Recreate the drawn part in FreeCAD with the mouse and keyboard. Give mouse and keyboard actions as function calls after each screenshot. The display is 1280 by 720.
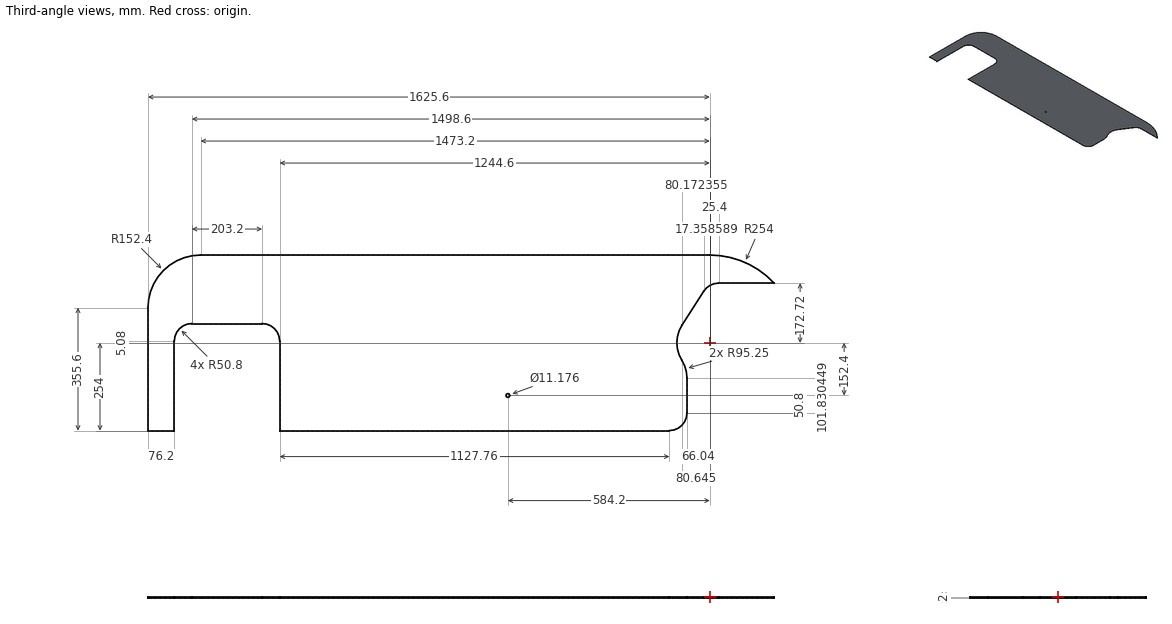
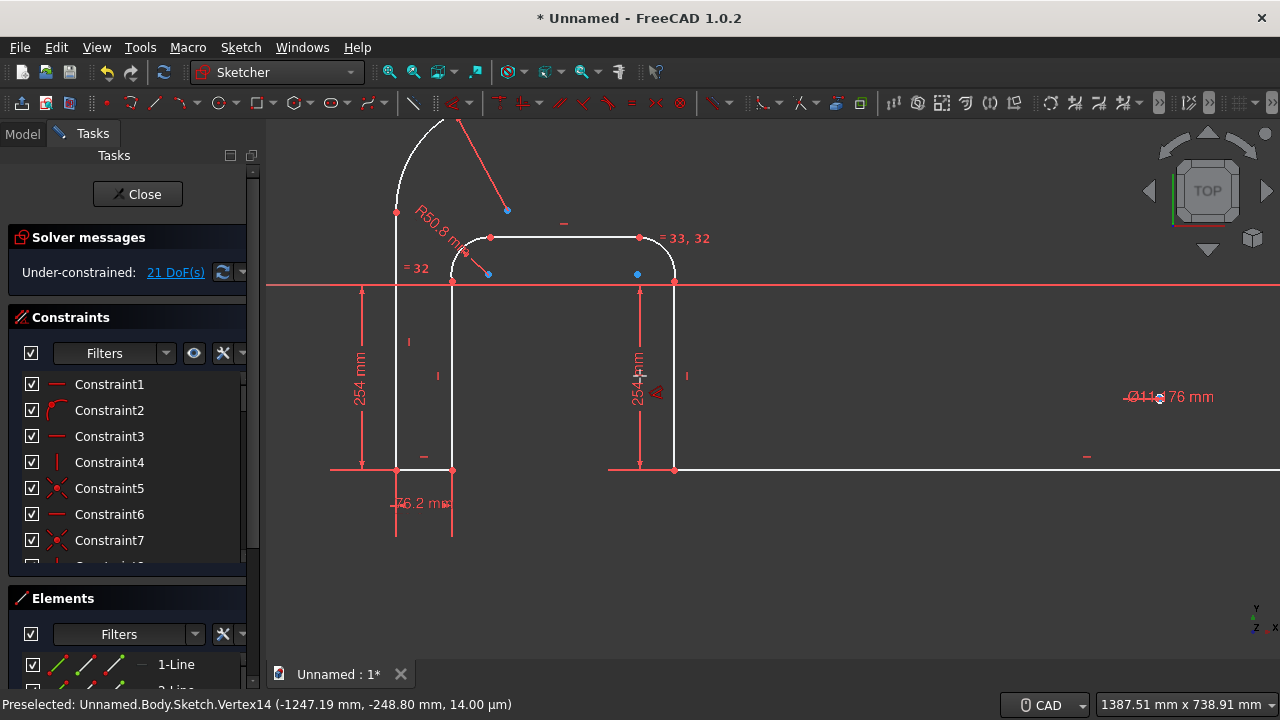
click(396, 393)
click(362, 341)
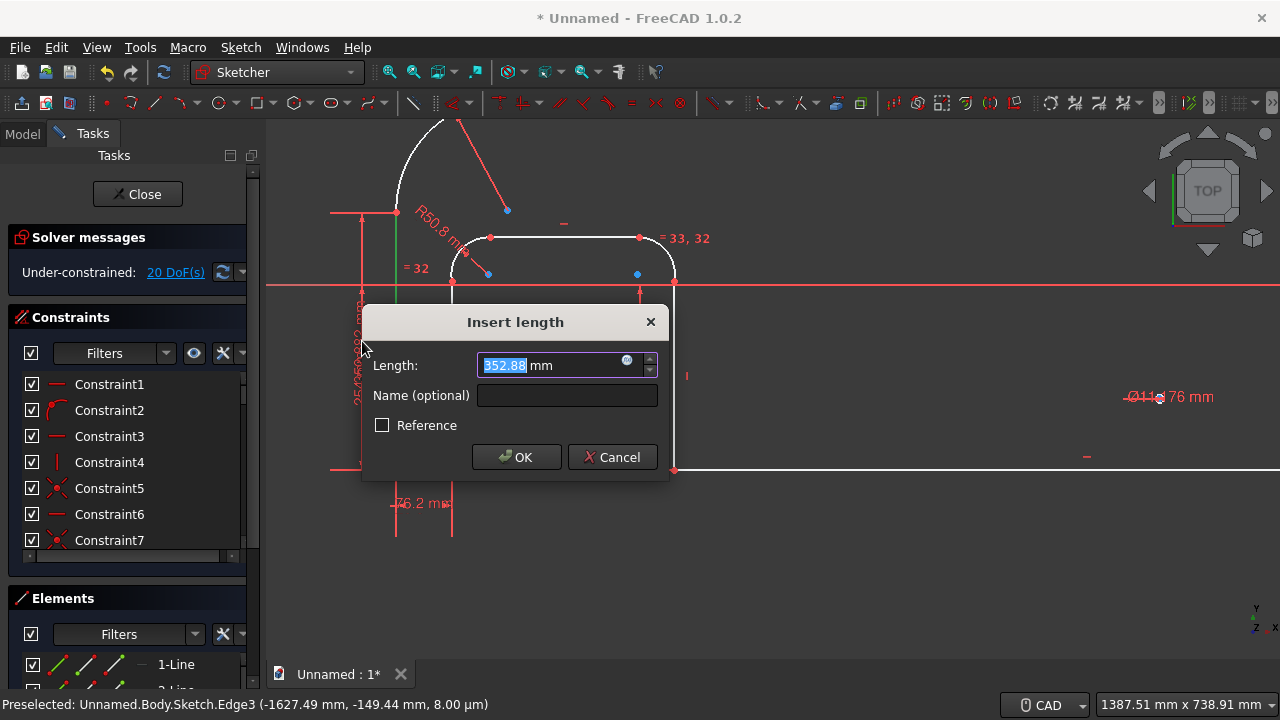
text(355.6)
key(Return)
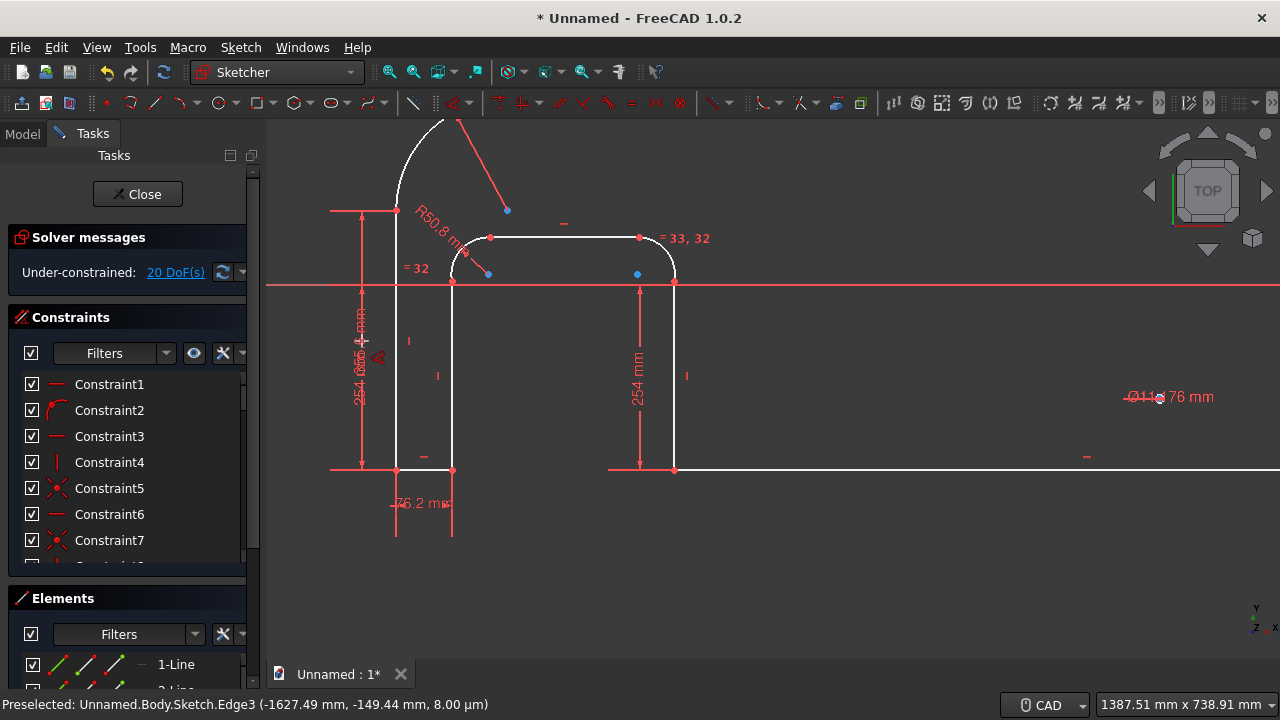
click(535, 237)
click(565, 203)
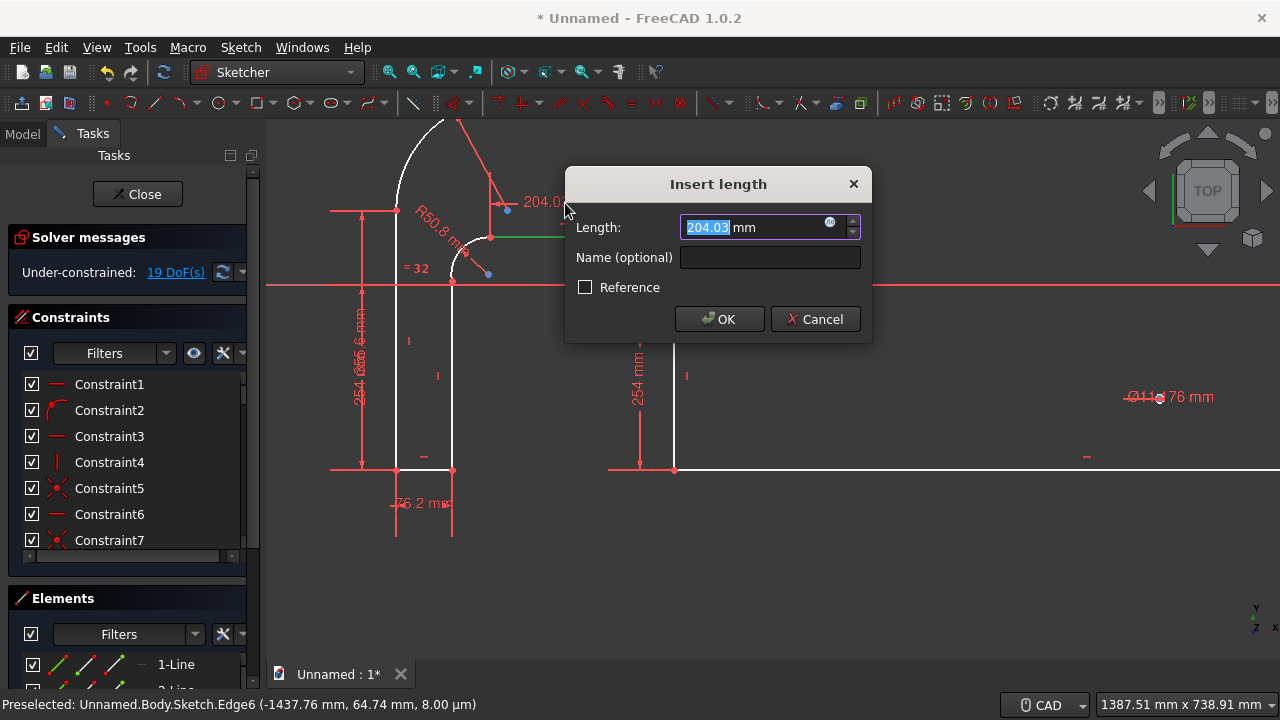
text(203.2)
key(Return)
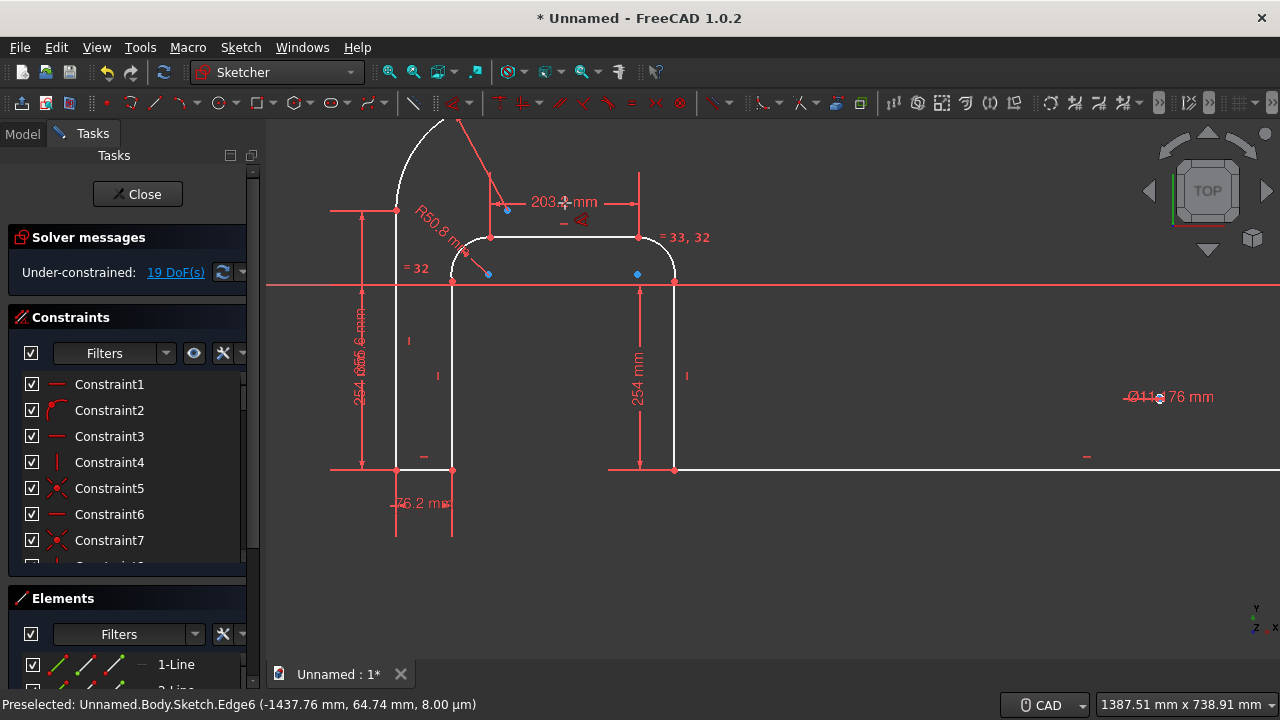
scroll(415, 474, down, 4)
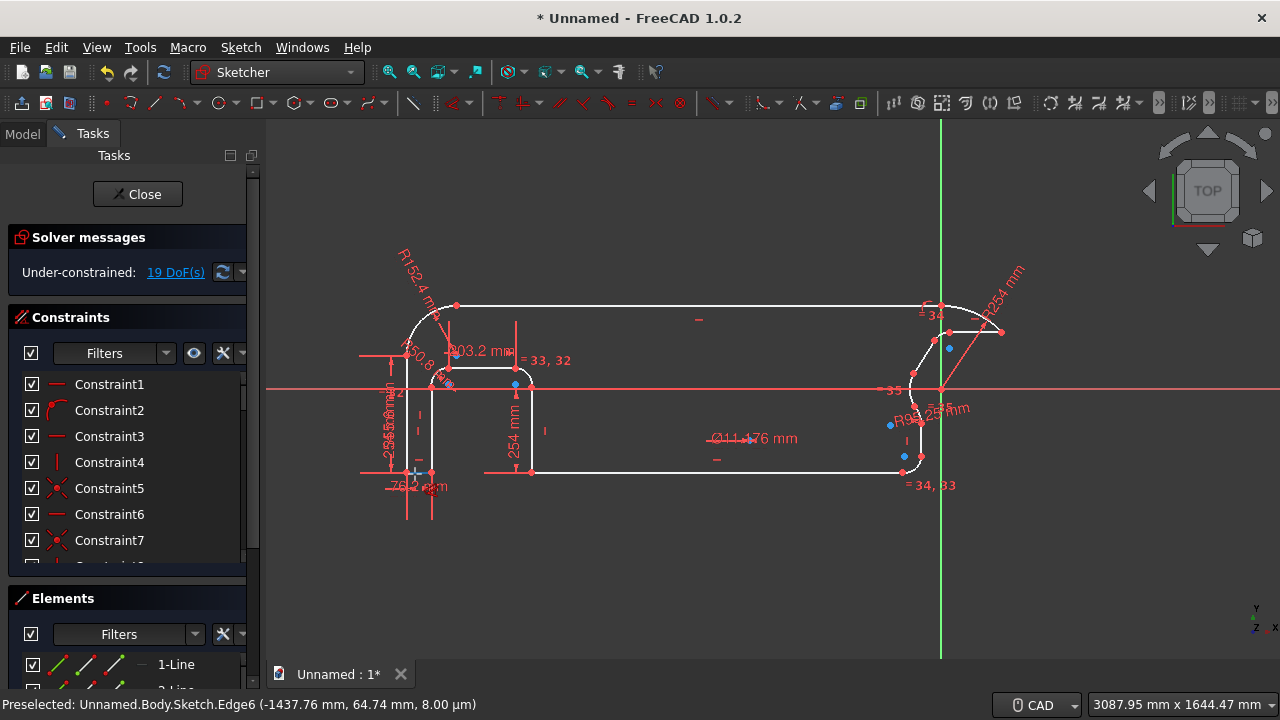
scroll(949, 332, up, 8)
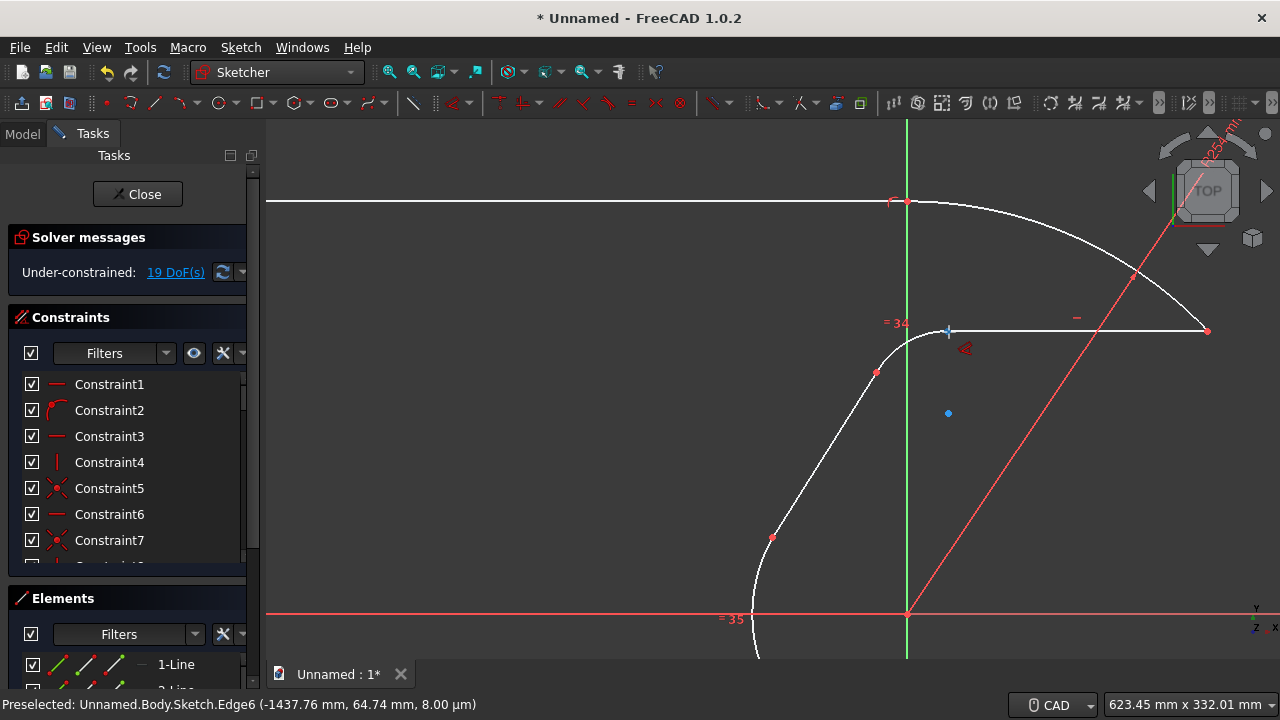
click(948, 331)
click(928, 297)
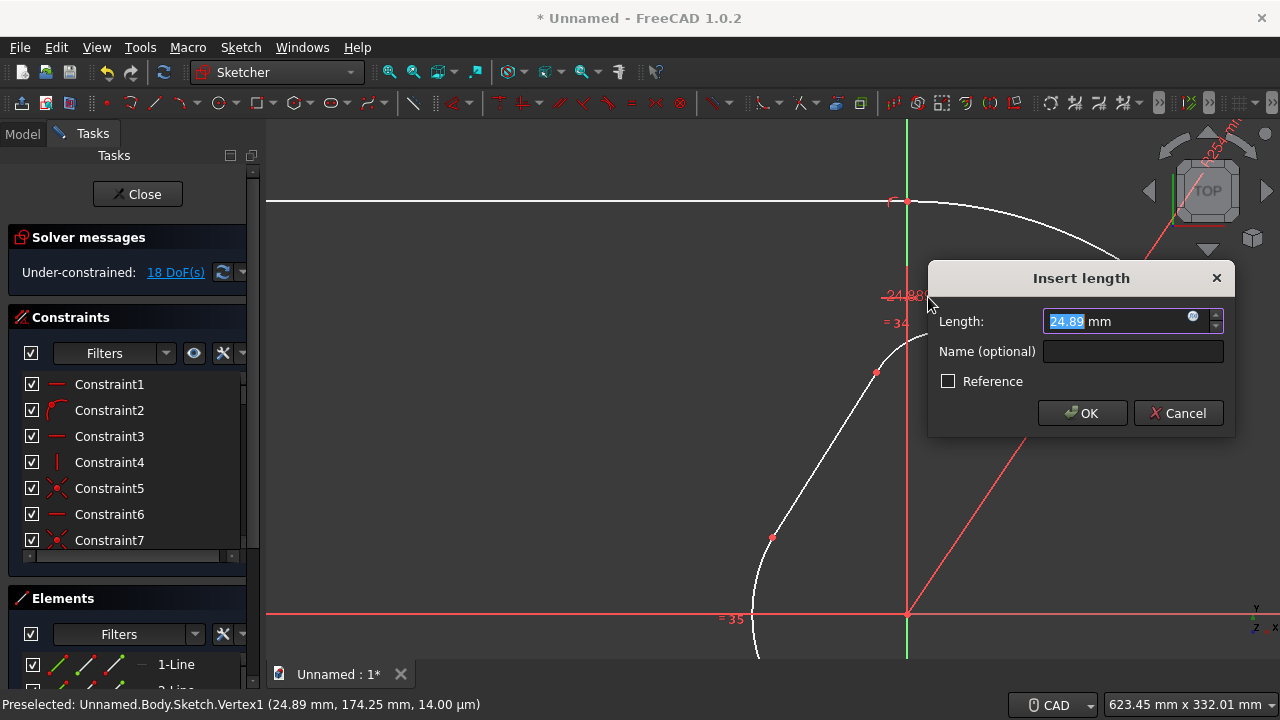
text(25.4)
key(Return)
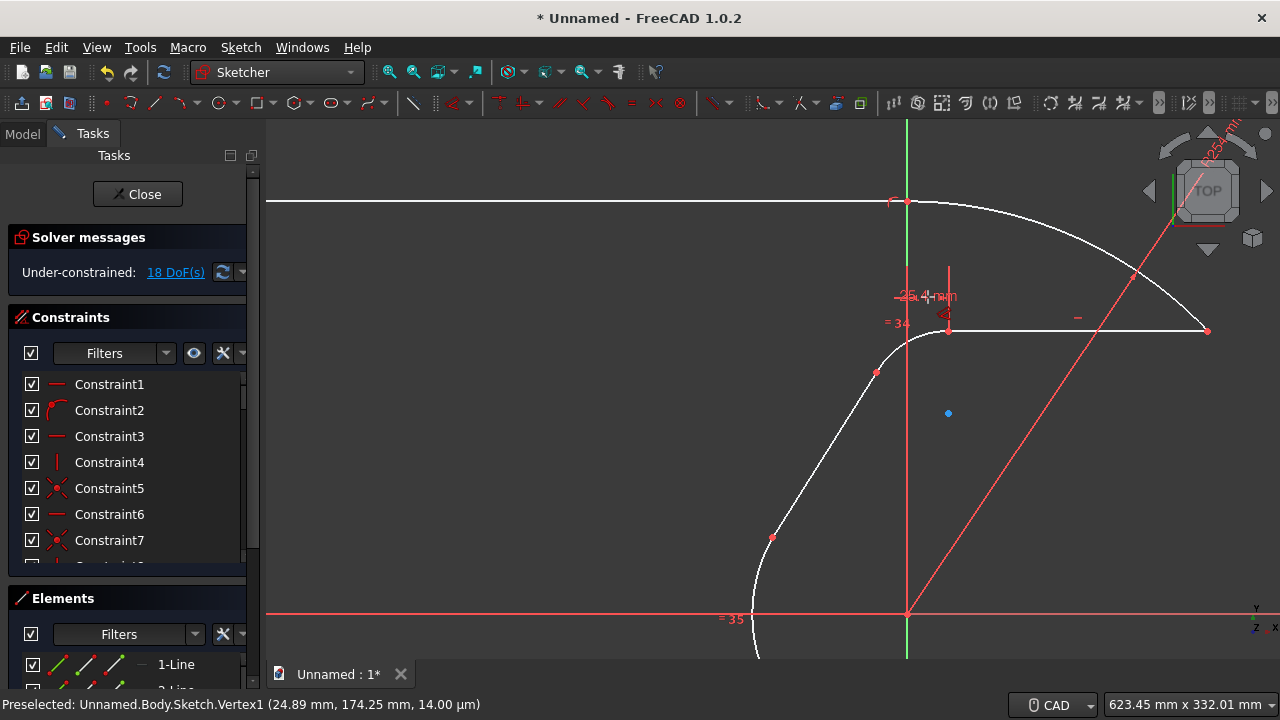
scroll(949, 332, down, 8)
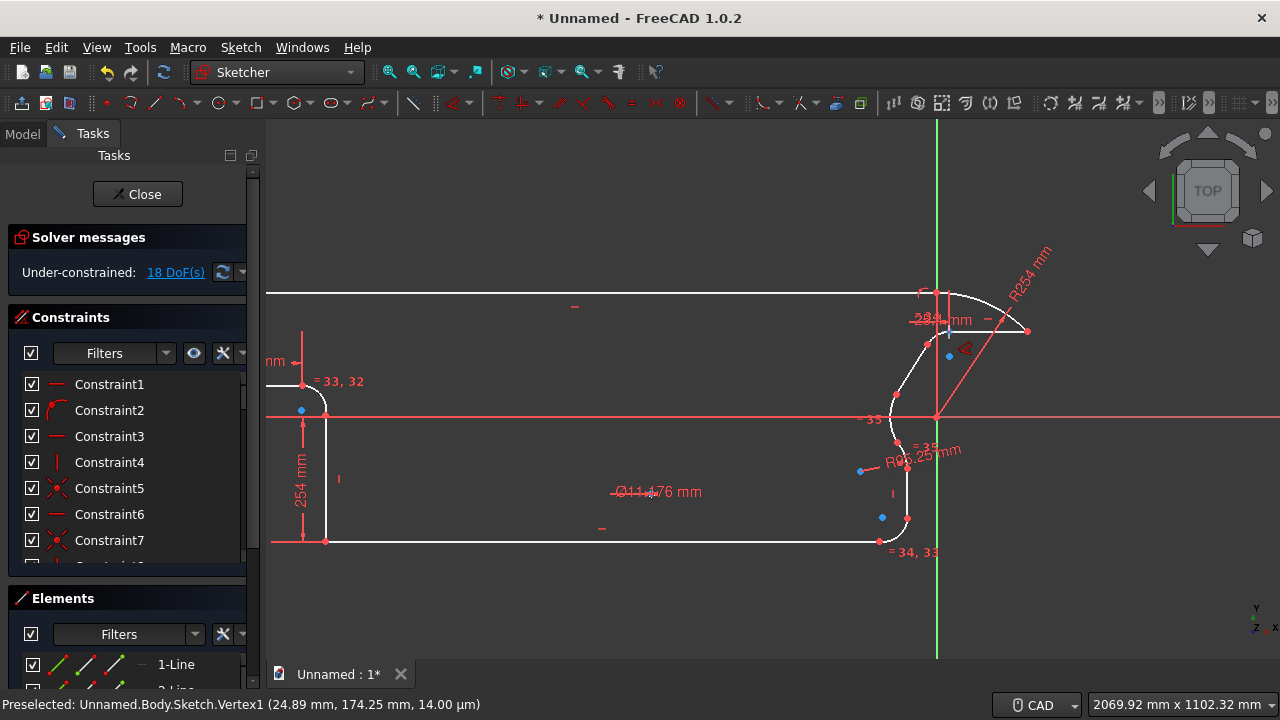
scroll(432, 388, up, 16)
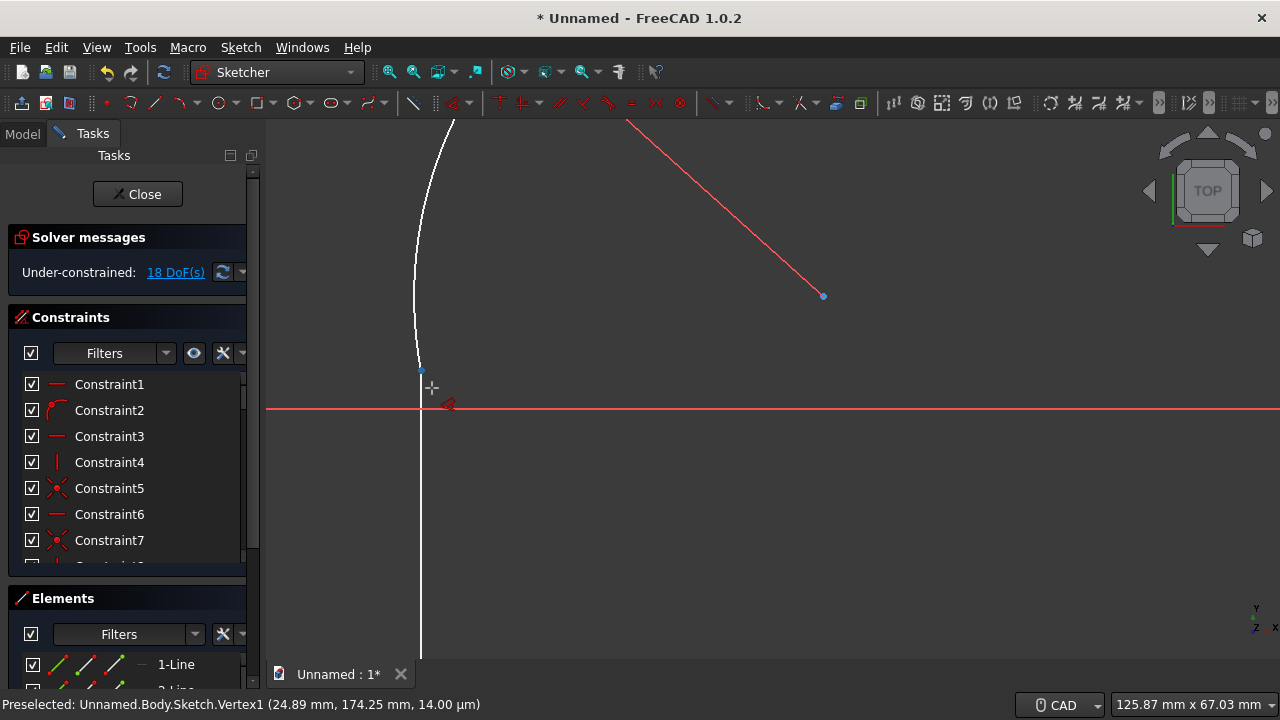
click(421, 371)
click(387, 390)